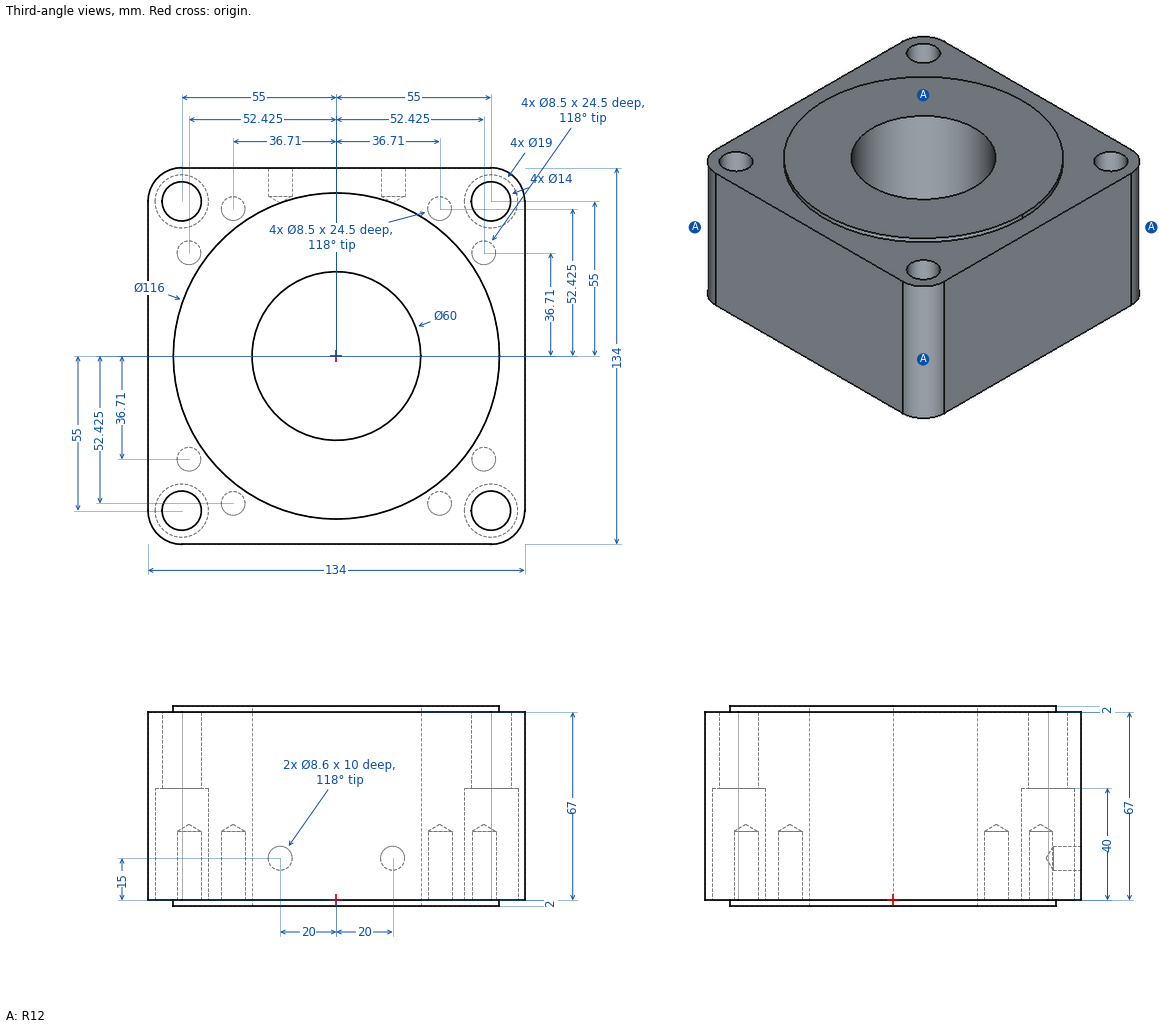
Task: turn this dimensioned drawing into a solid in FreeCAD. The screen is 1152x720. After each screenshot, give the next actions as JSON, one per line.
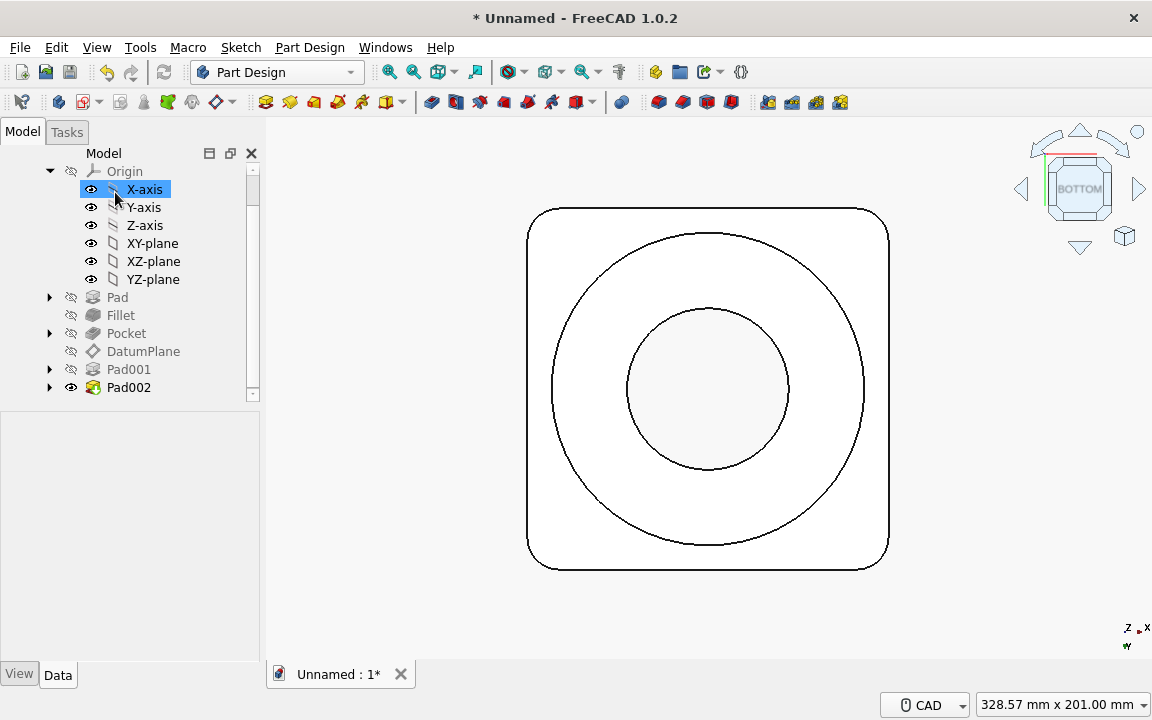
{"action": "left_click", "coordinate": [84, 102]}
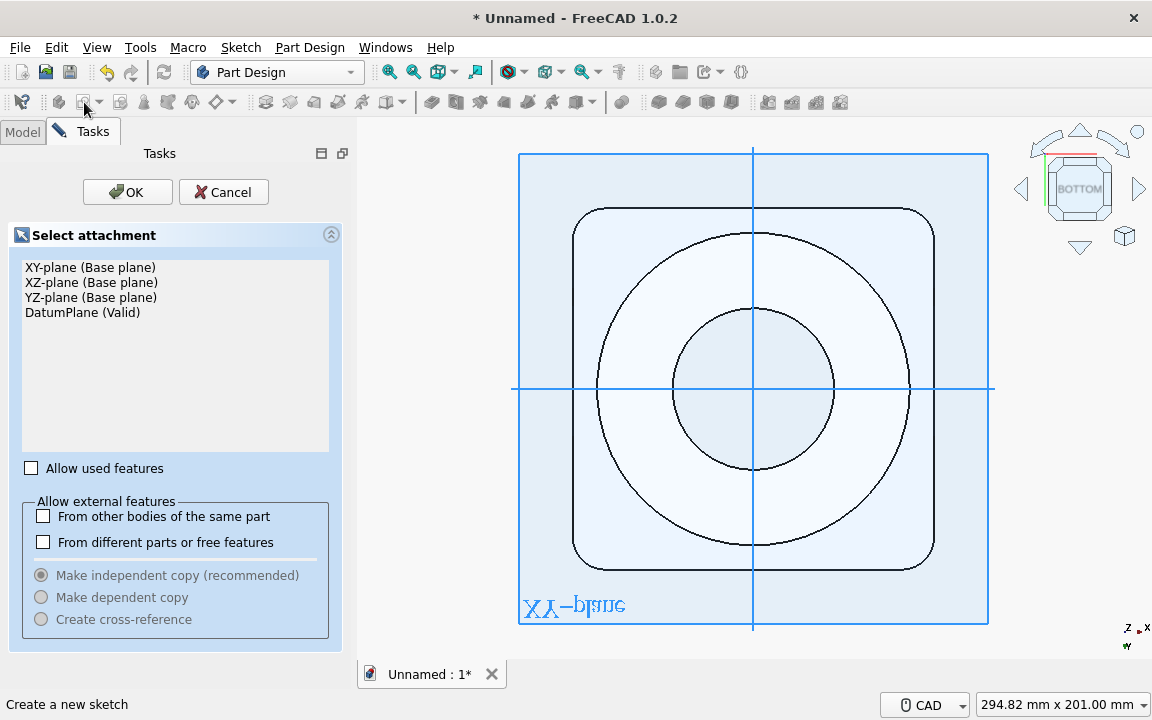
{"action": "left_click", "coordinate": [82, 268]}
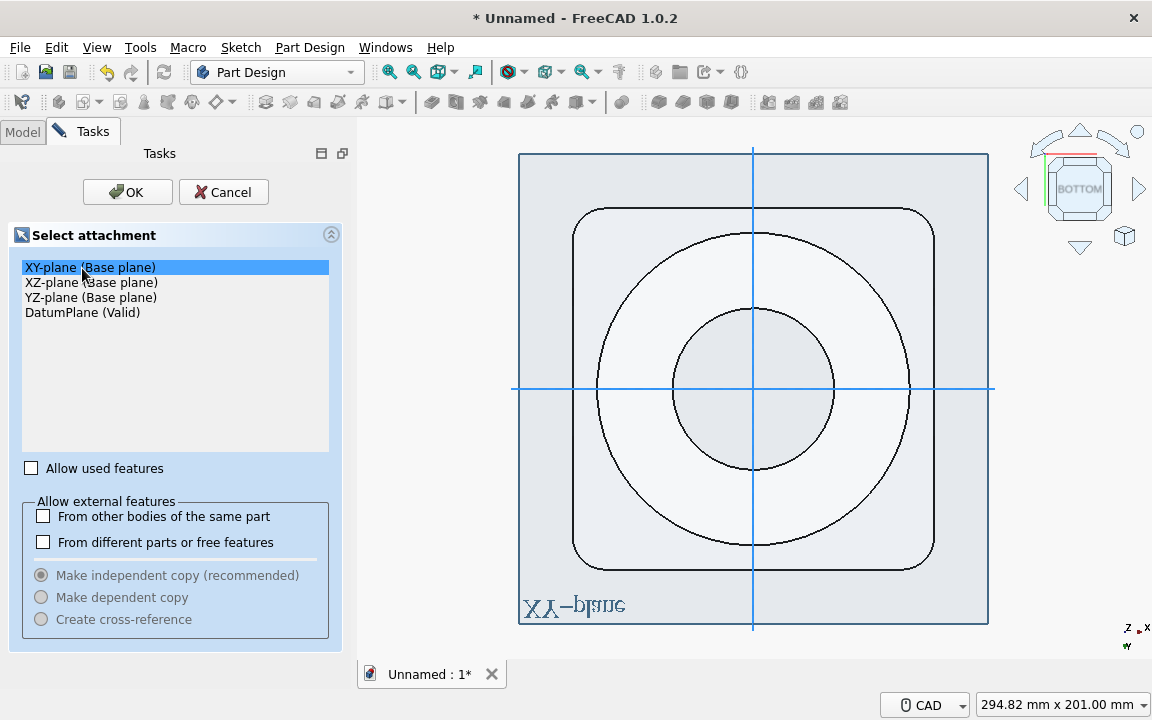
{"action": "left_click", "coordinate": [128, 192]}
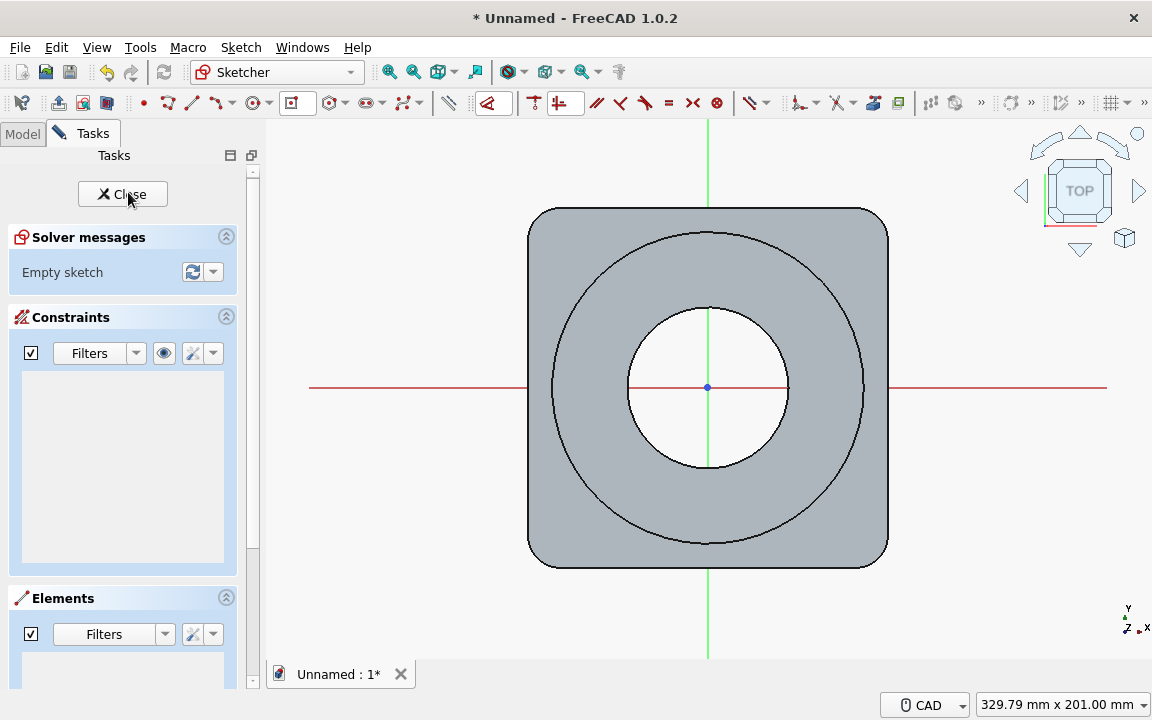
{"action": "left_click", "coordinate": [108, 104]}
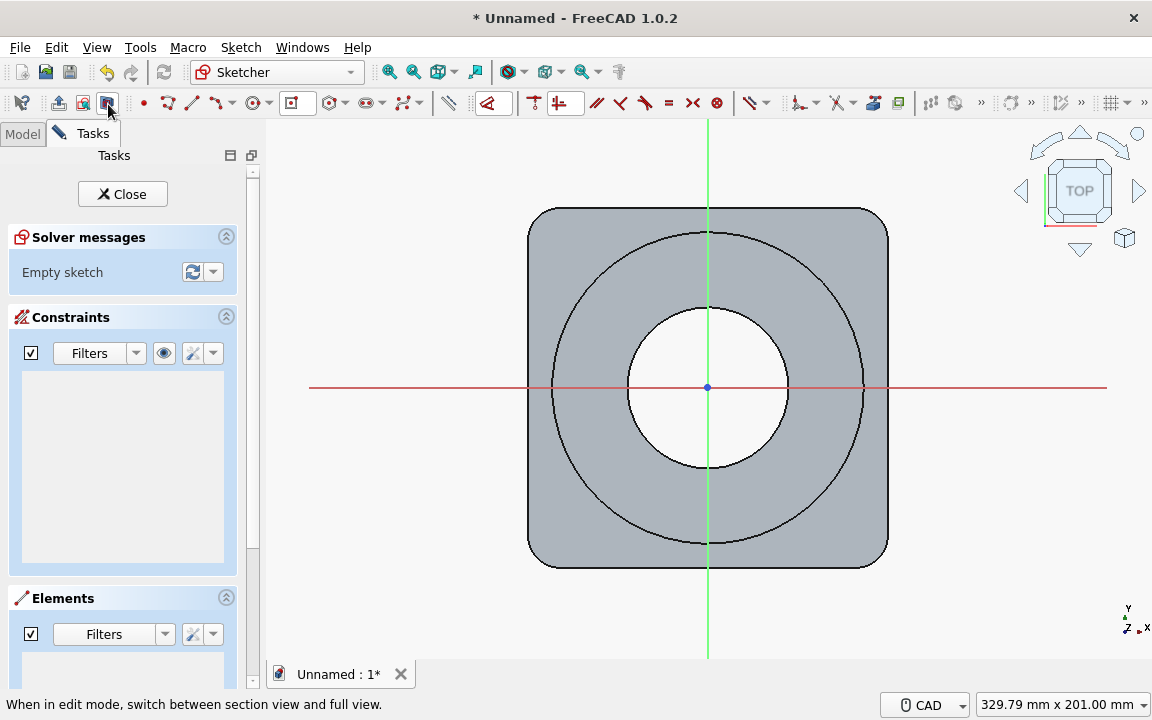
{"action": "left_click", "coordinate": [254, 104]}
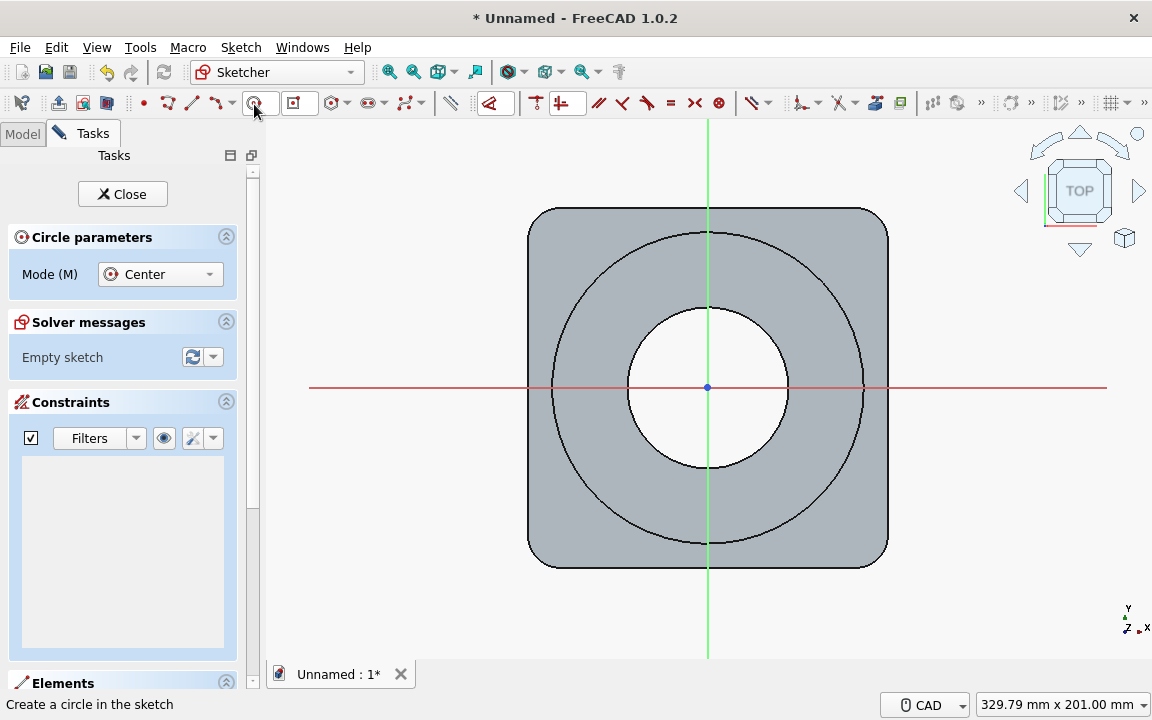
{"action": "left_click", "coordinate": [856, 240]}
{"action": "left_click", "coordinate": [869, 227]}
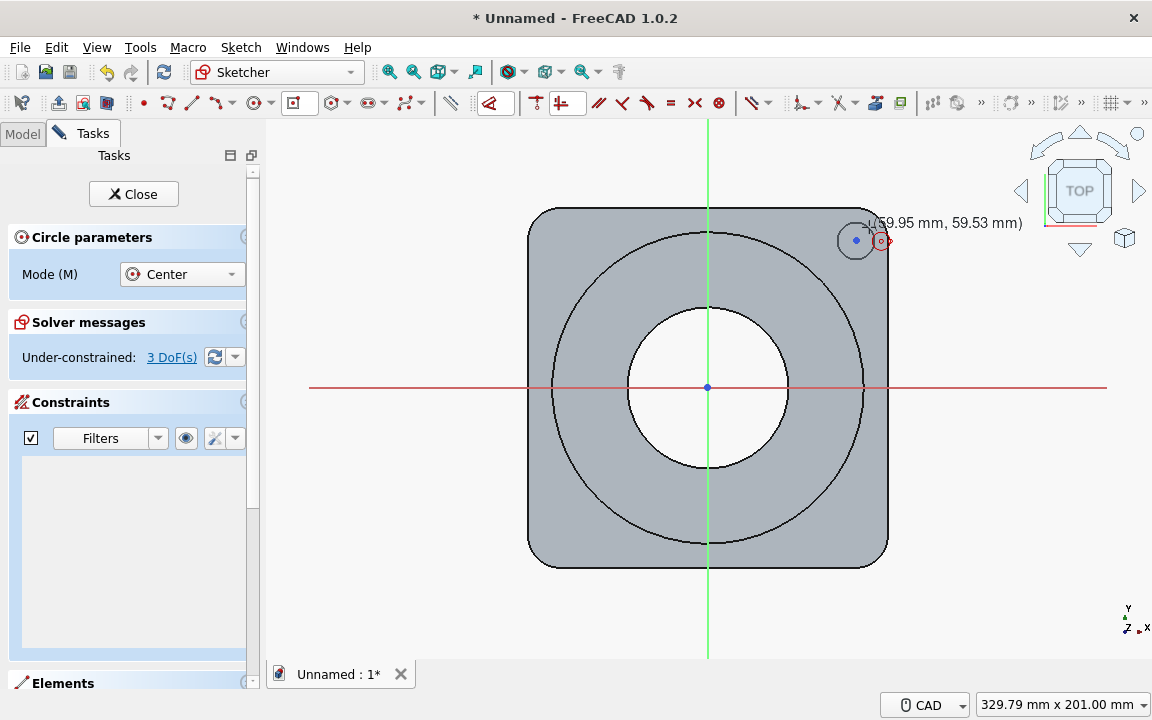
{"action": "left_click", "coordinate": [560, 240]}
{"action": "left_click", "coordinate": [573, 227]}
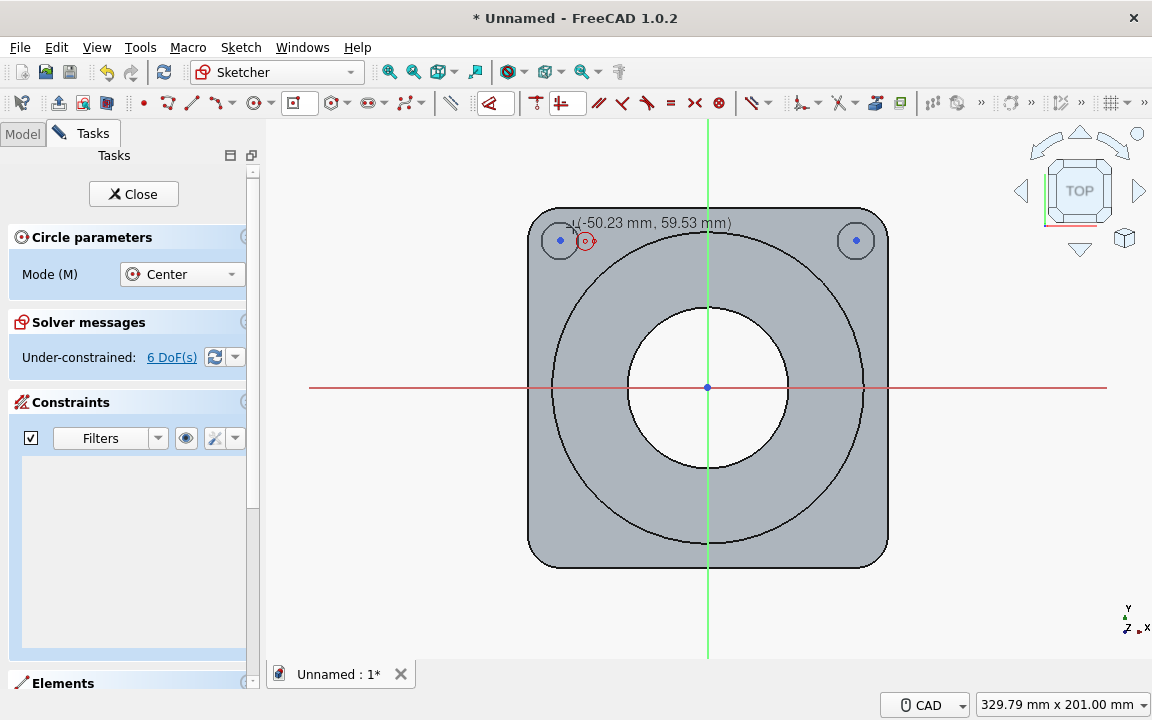
{"action": "left_click", "coordinate": [560, 536]}
{"action": "left_click", "coordinate": [573, 522]}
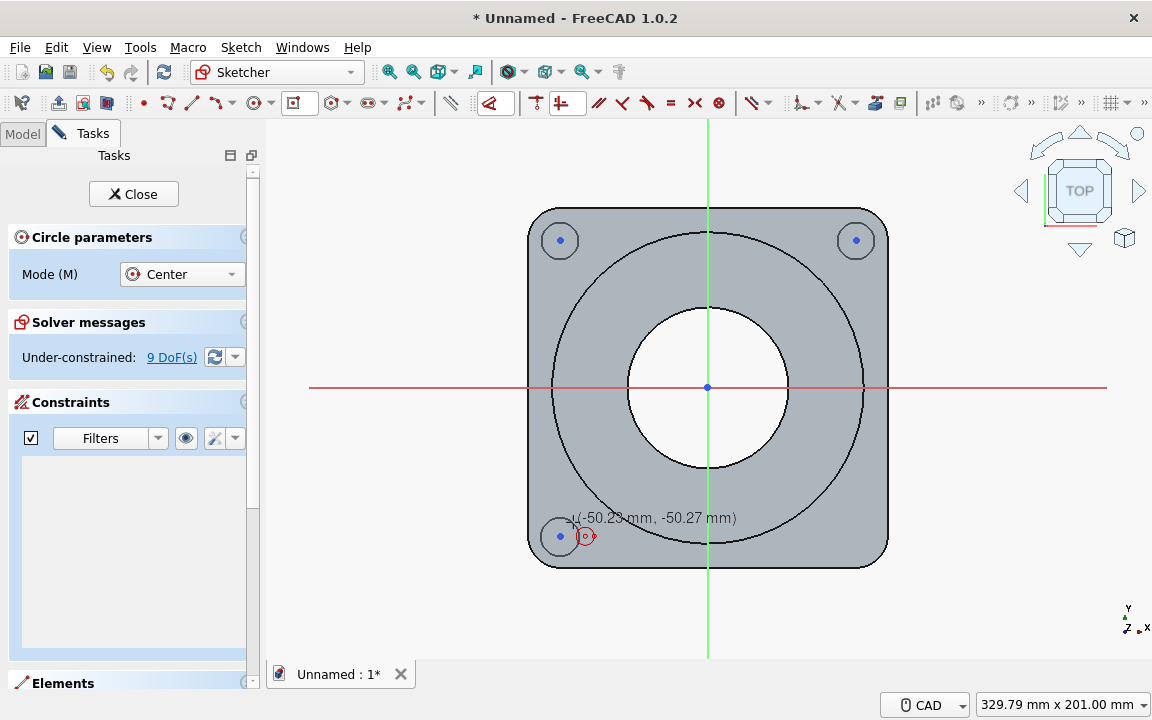
{"action": "left_click", "coordinate": [856, 536]}
{"action": "left_click", "coordinate": [869, 522]}
{"action": "key", "text": "Escape"}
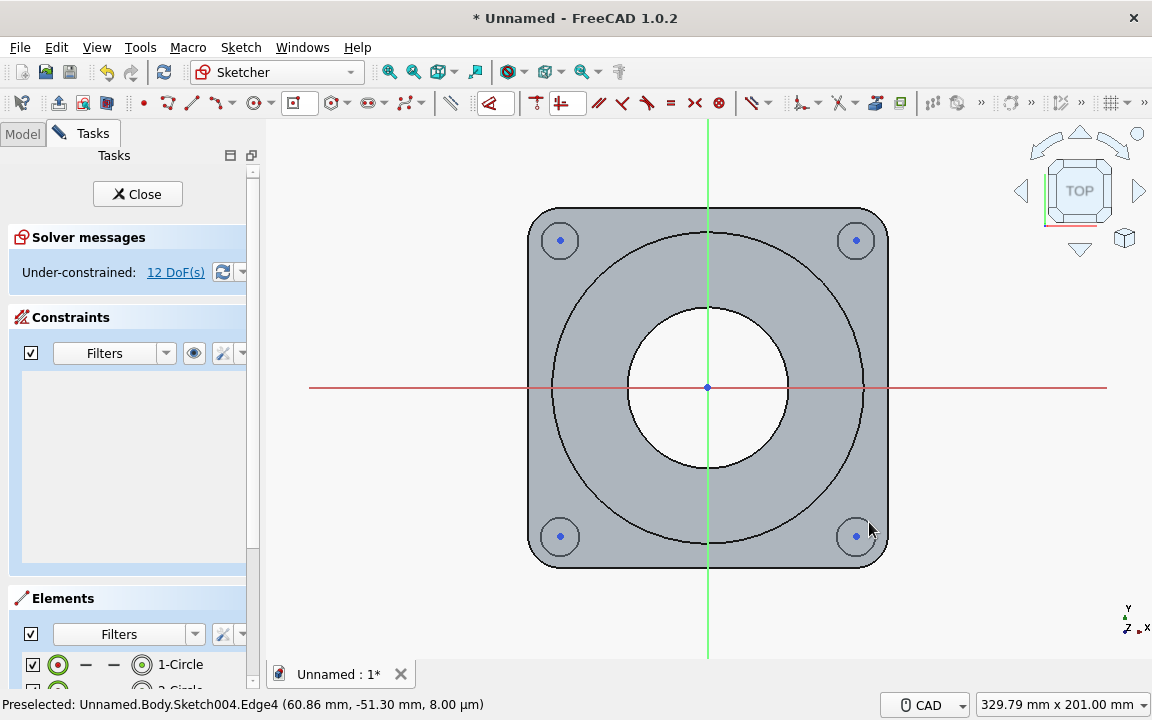
{"action": "left_click", "coordinate": [869, 228]}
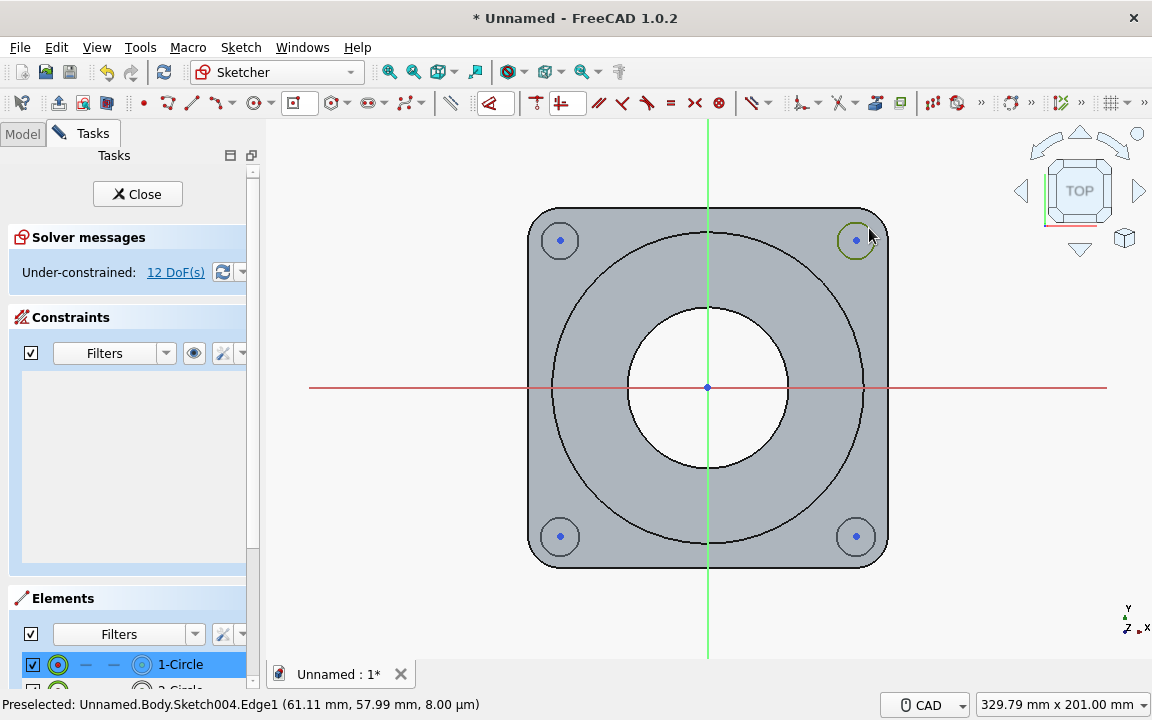
{"action": "left_click", "coordinate": [573, 228]}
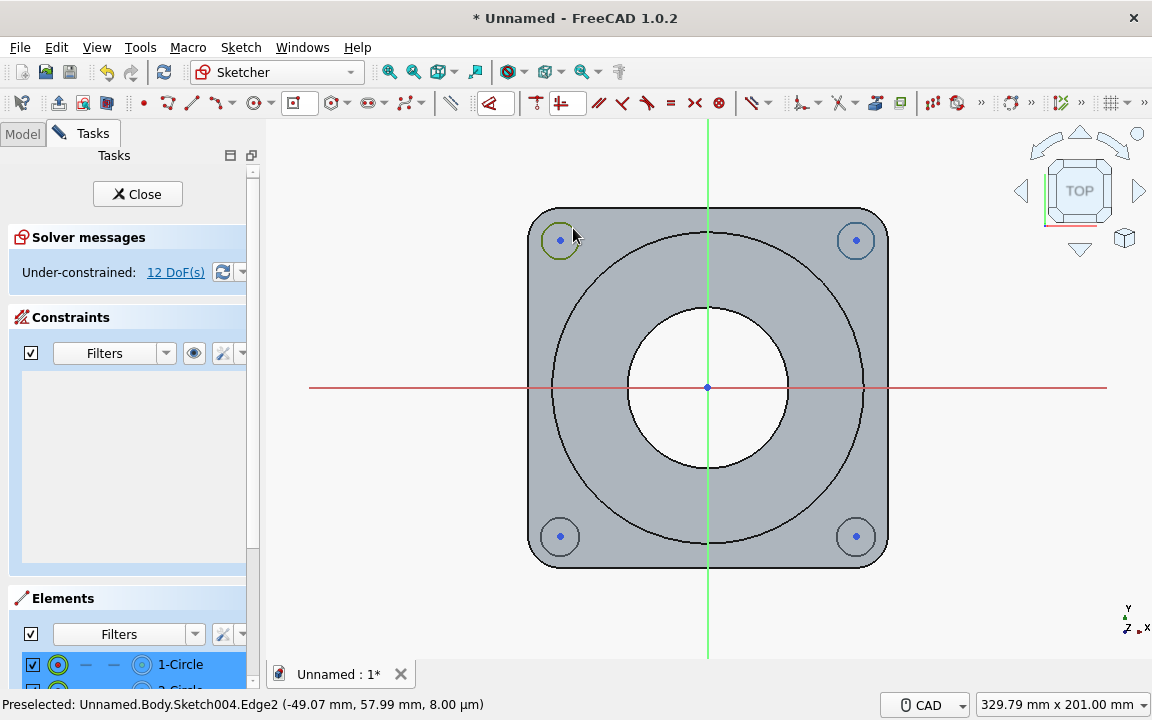
{"action": "left_click", "coordinate": [573, 523]}